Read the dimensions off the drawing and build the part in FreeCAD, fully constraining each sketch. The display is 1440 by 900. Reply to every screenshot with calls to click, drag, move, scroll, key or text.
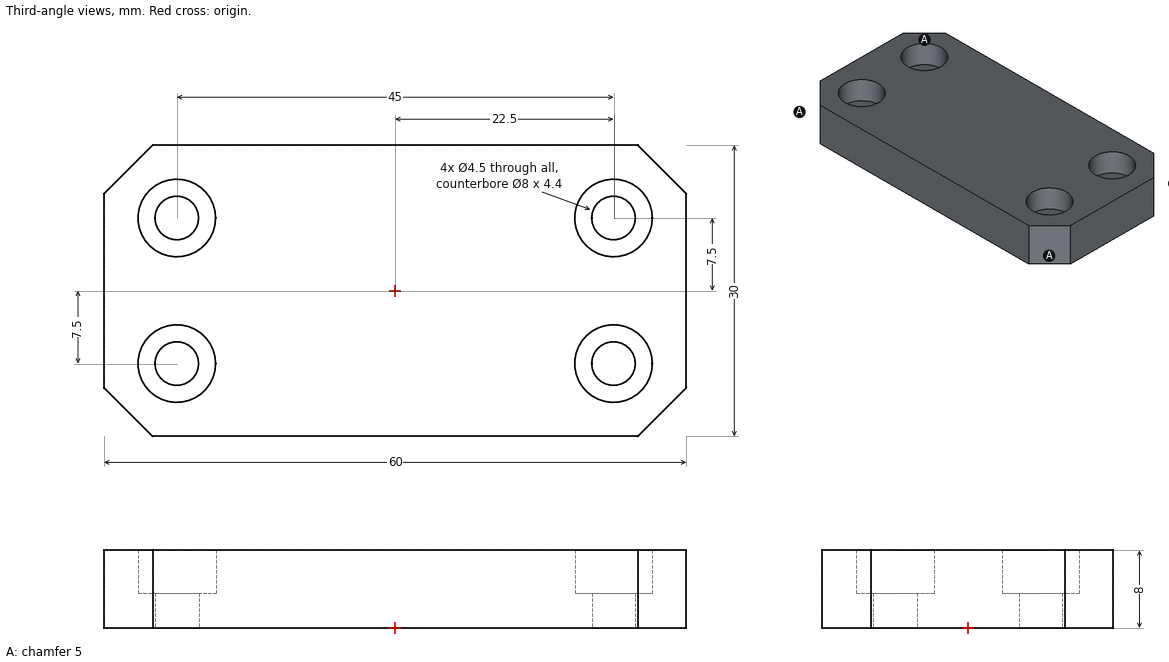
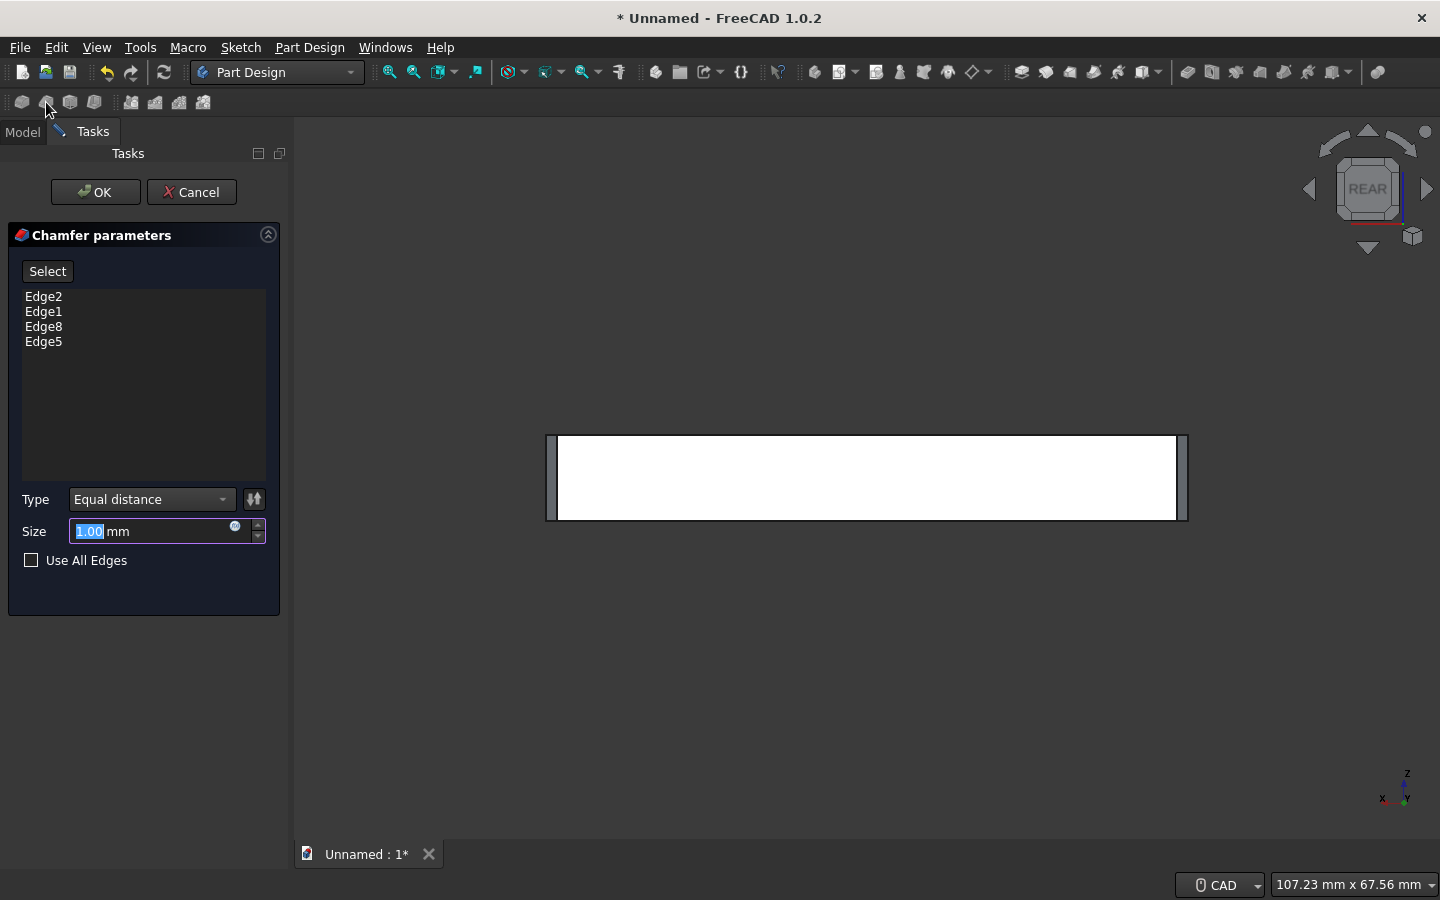
text(5)
key(Tab)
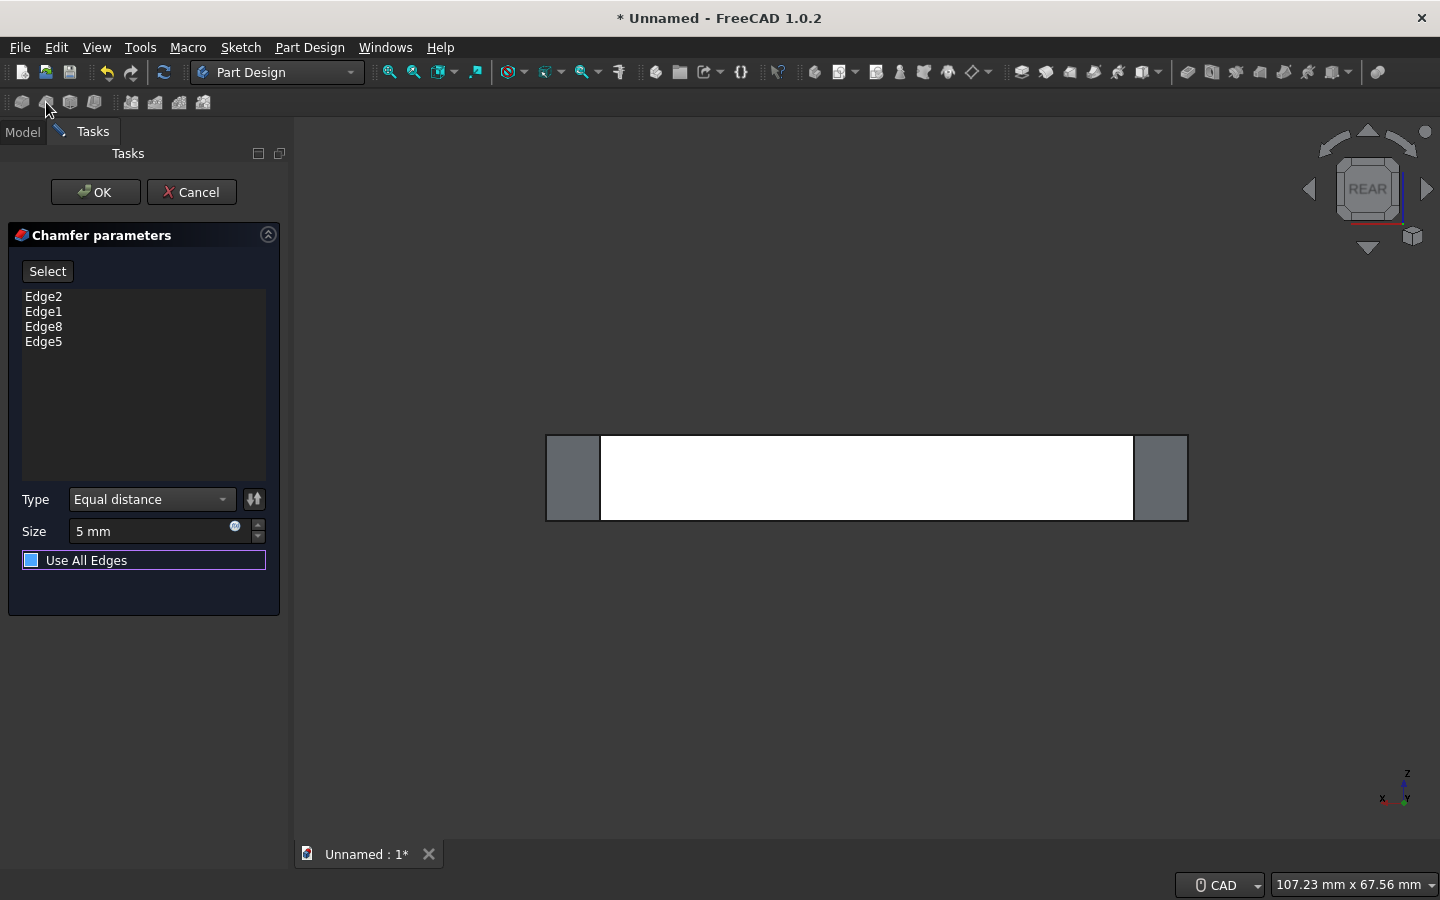
click(96, 192)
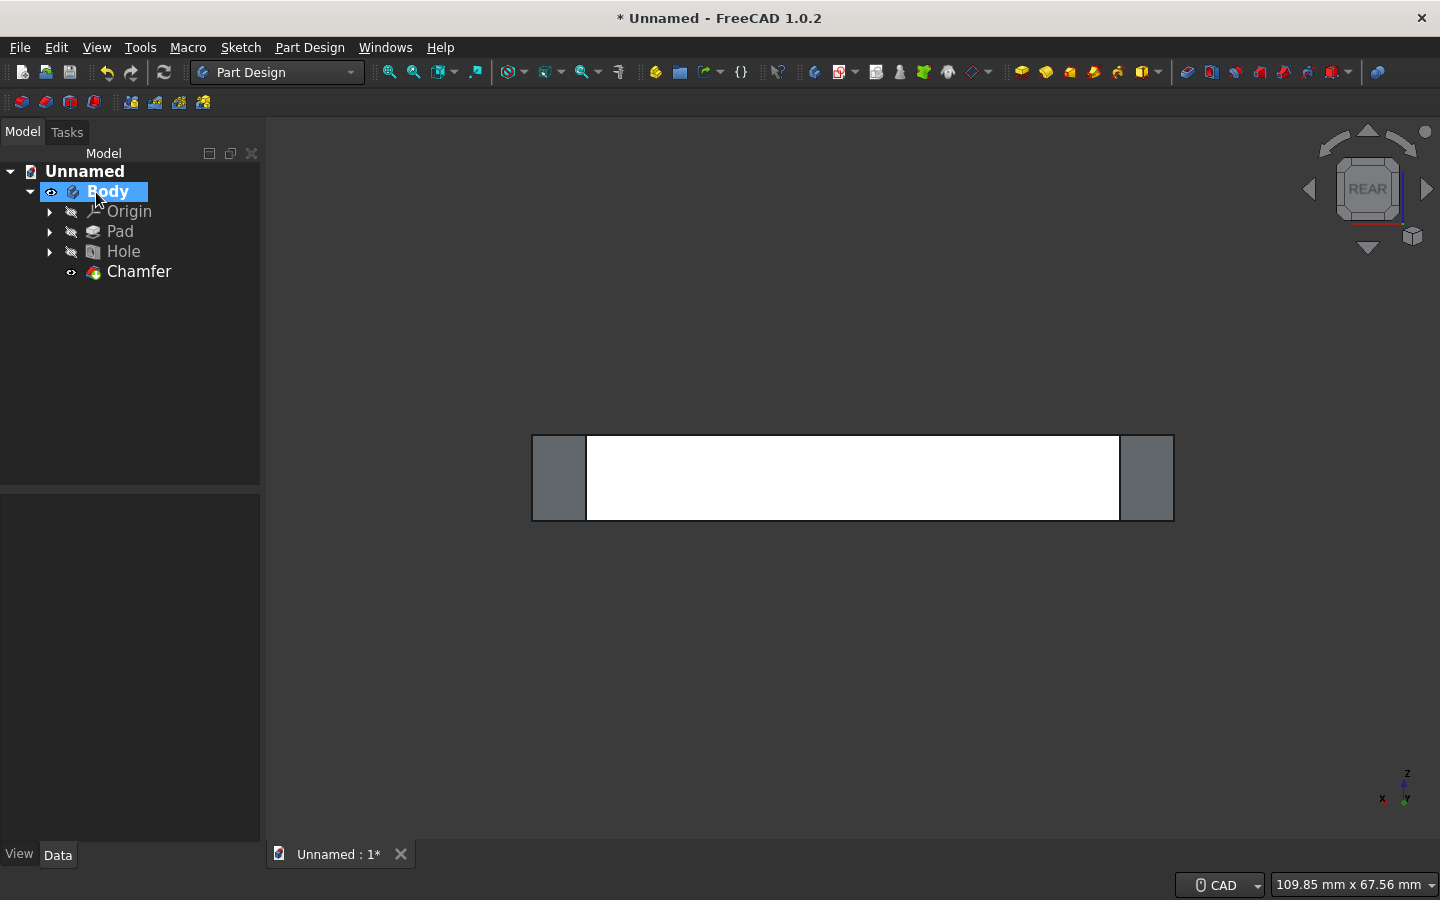
key(0)